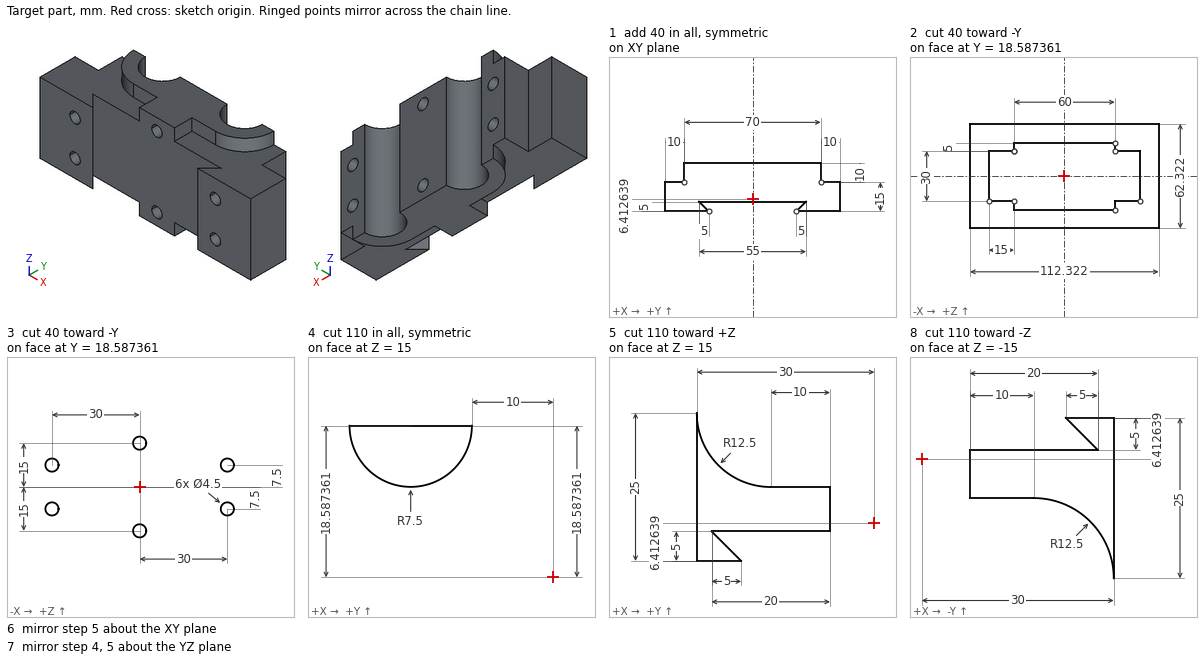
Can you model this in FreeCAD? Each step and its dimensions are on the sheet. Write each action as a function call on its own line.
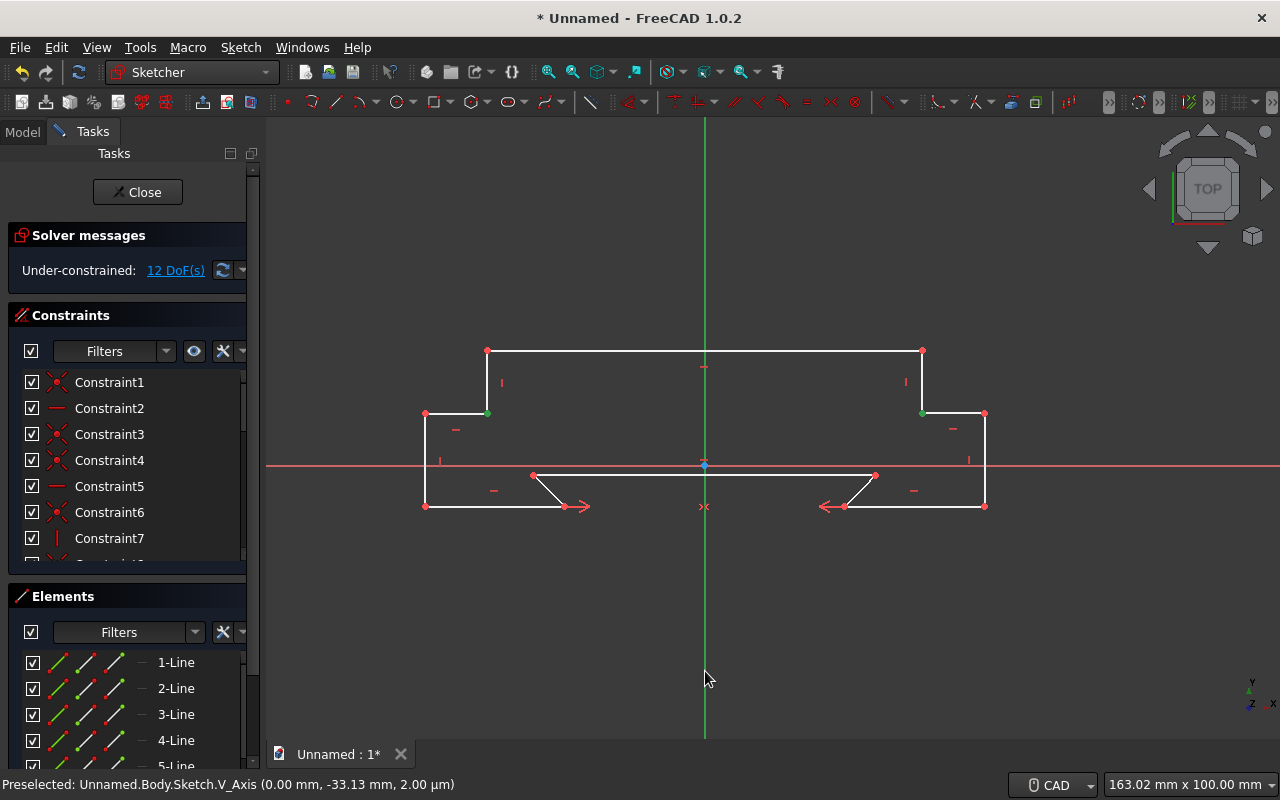
key(s)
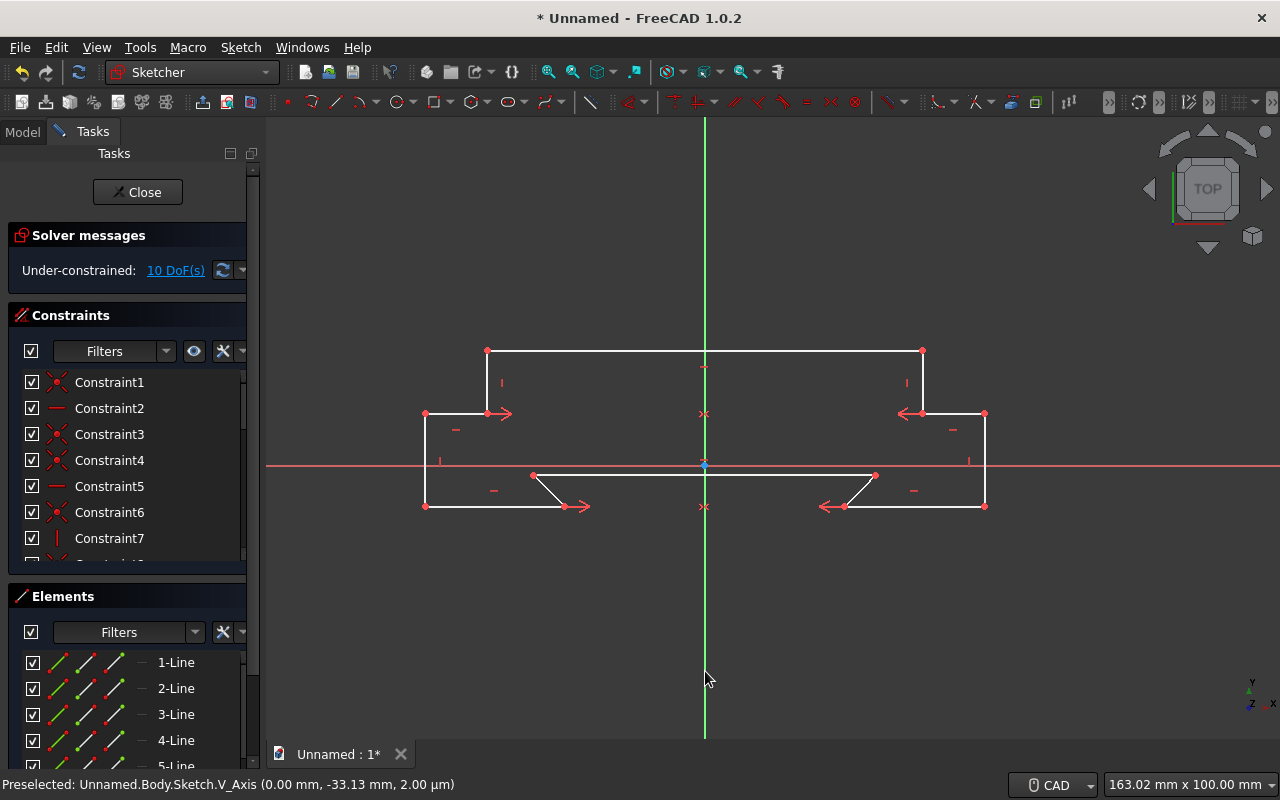
key(d)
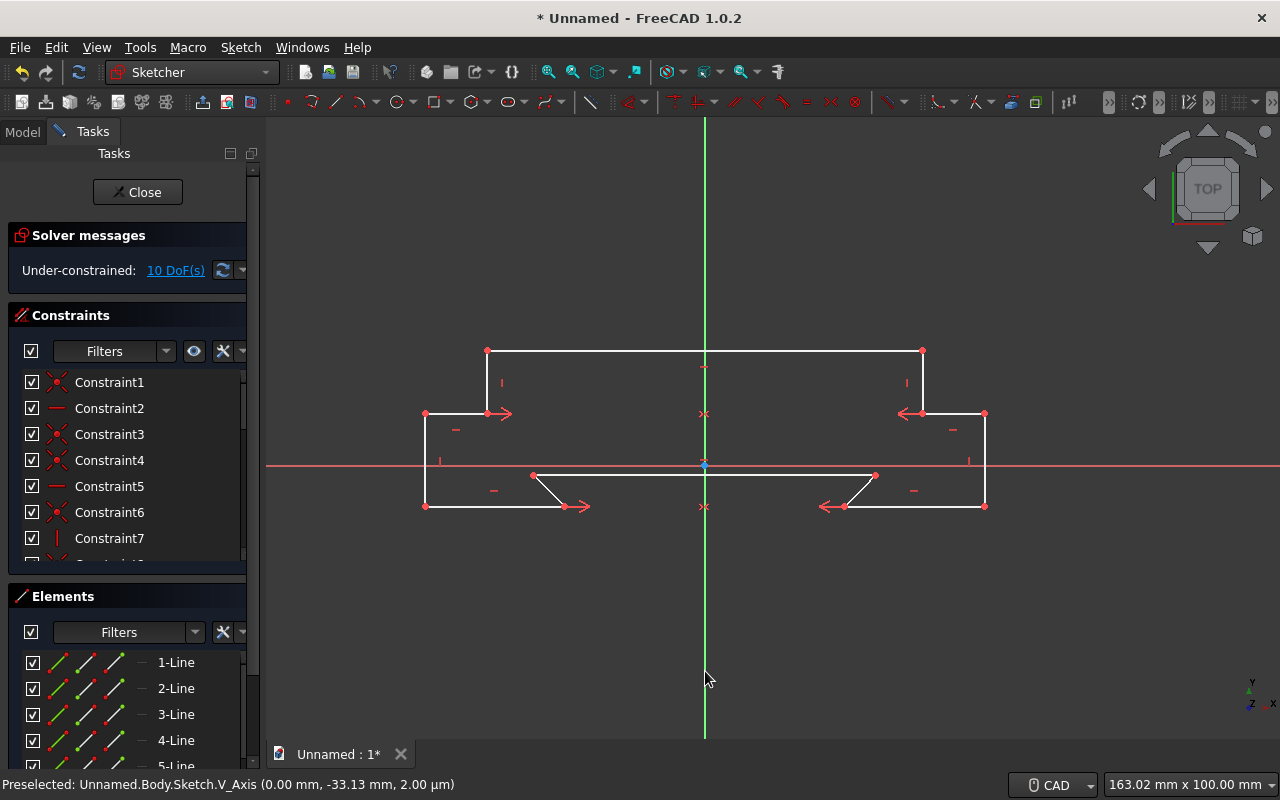
scroll(636, 475, up, 3)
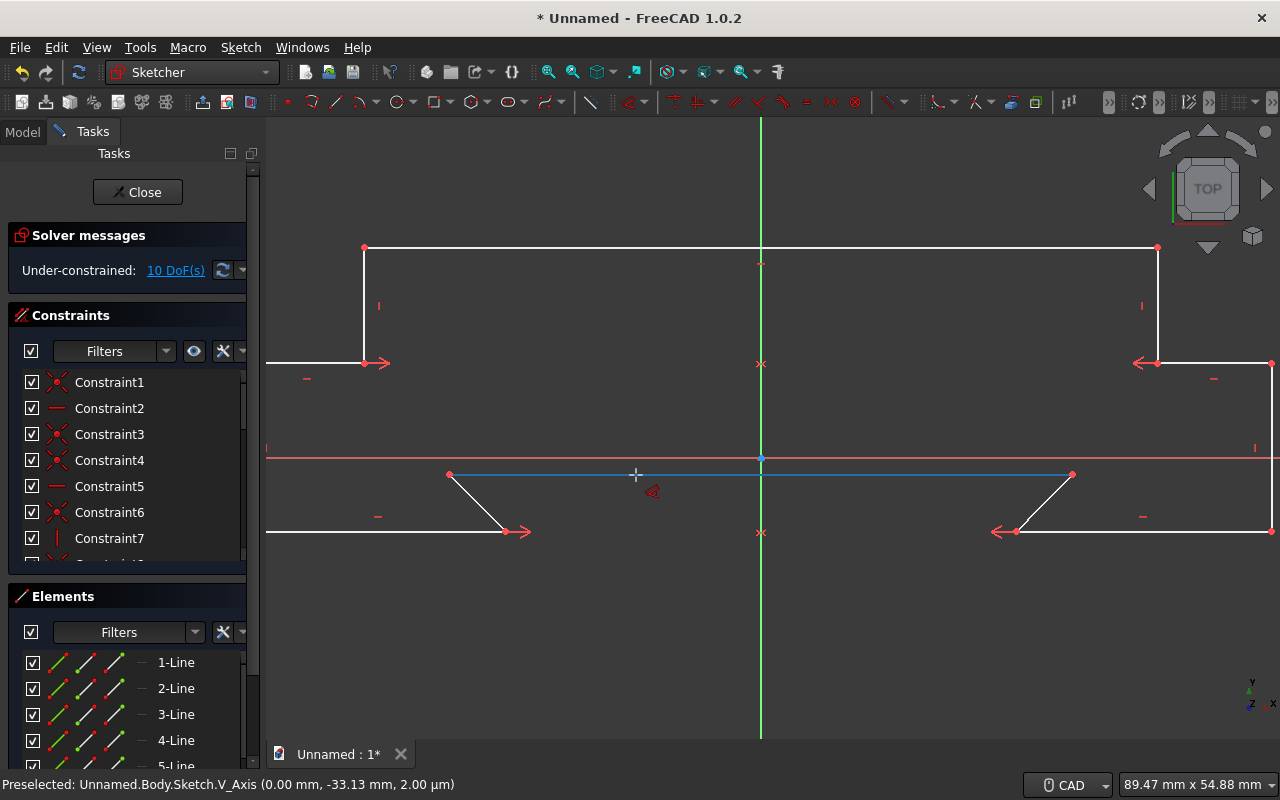
click(637, 475)
click(618, 509)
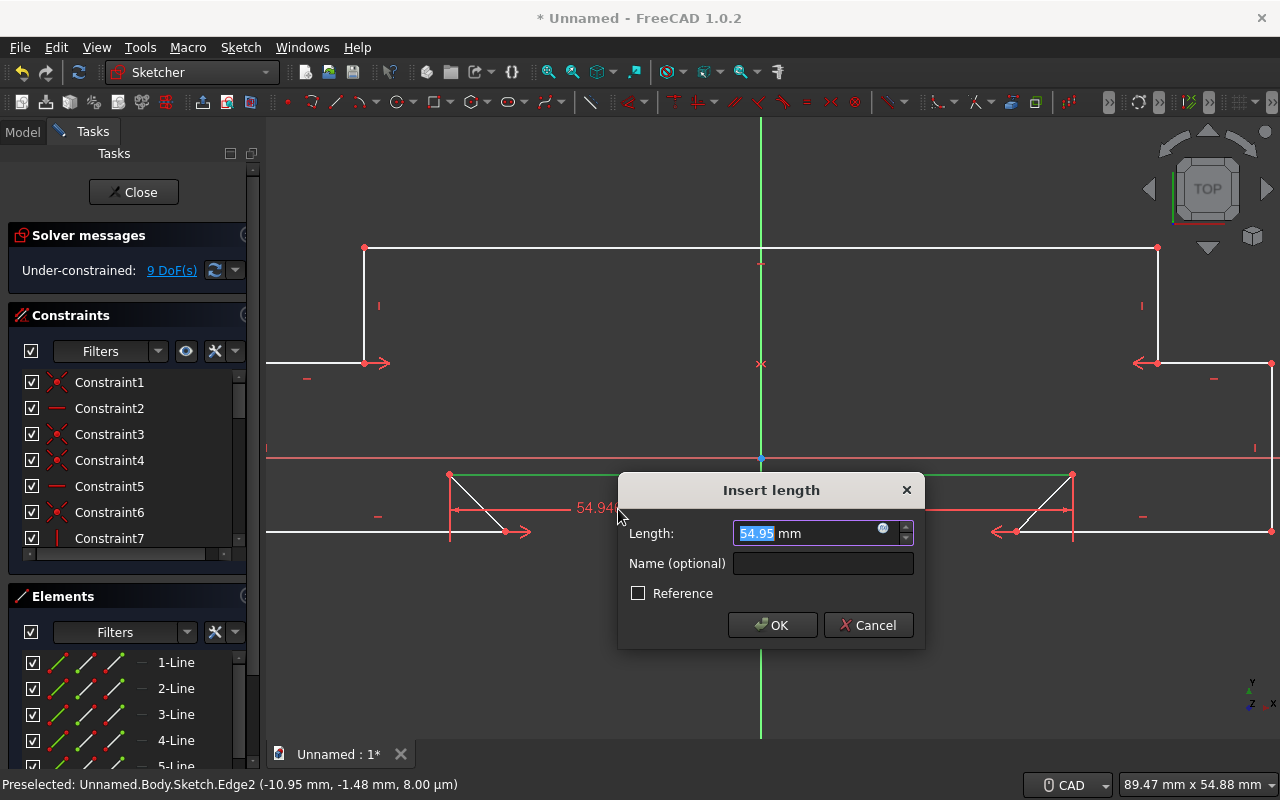
text(55)
key(Return)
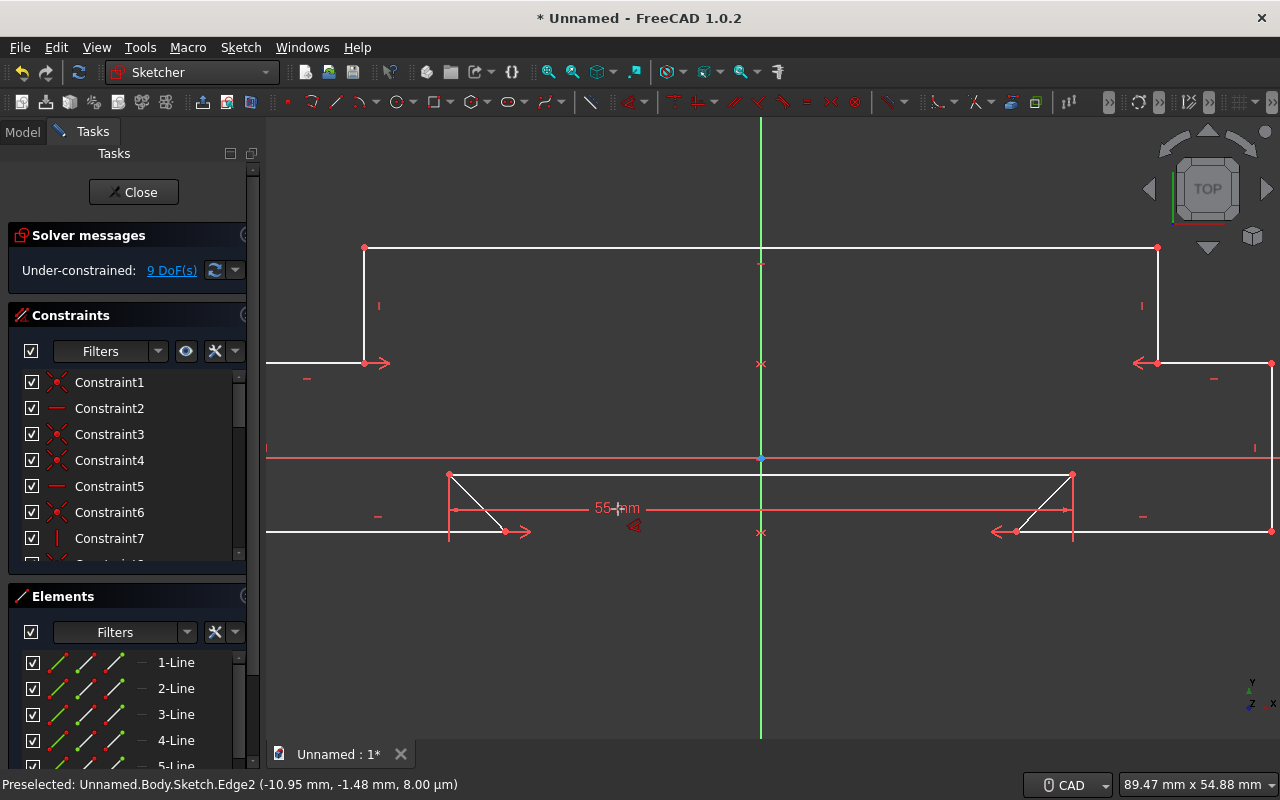
scroll(636, 475, down, 3)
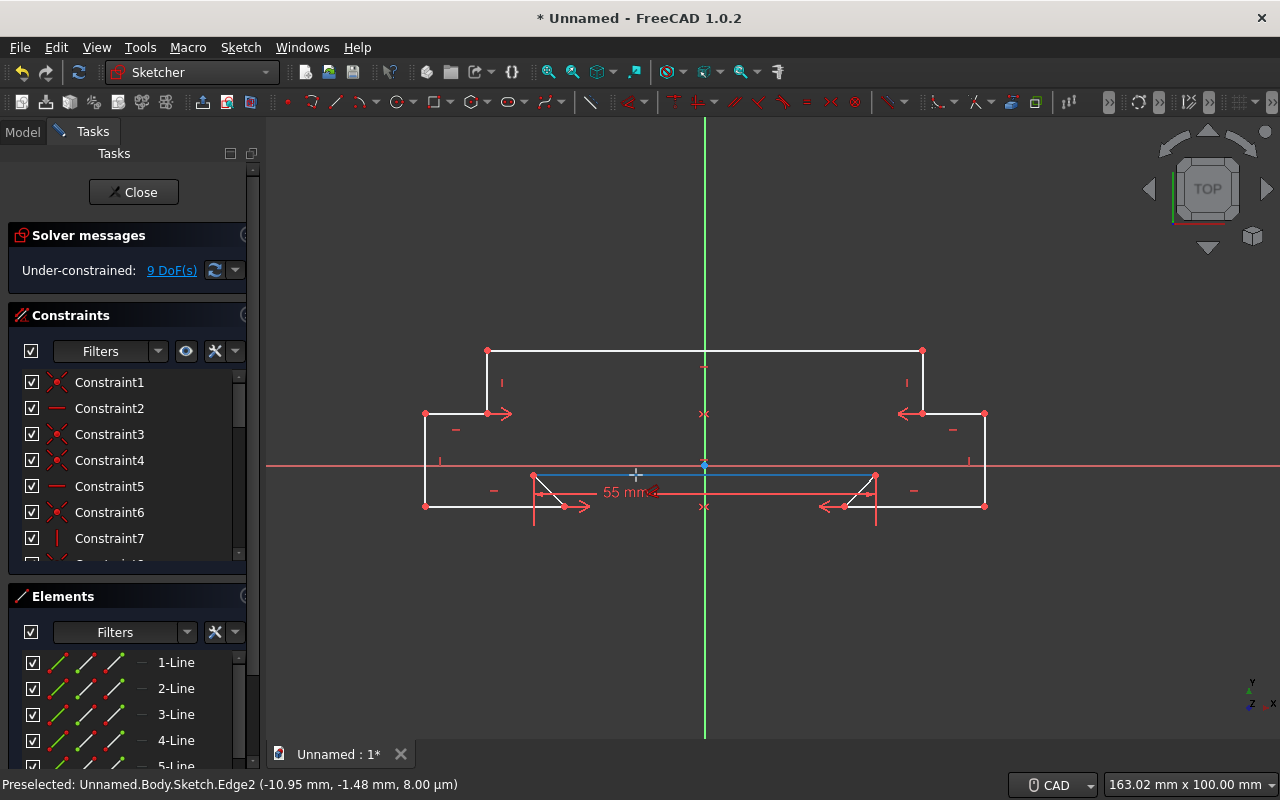
click(985, 479)
click(1019, 439)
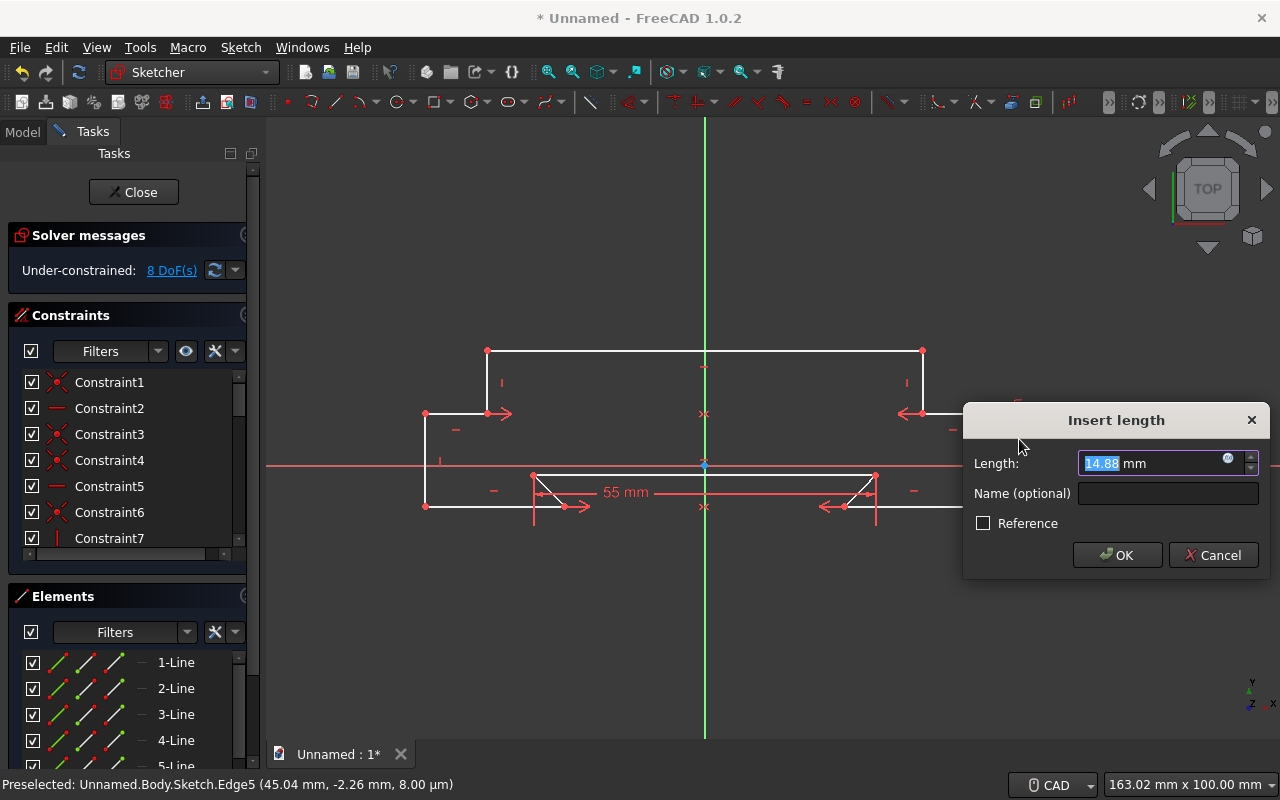
text(15)
key(Return)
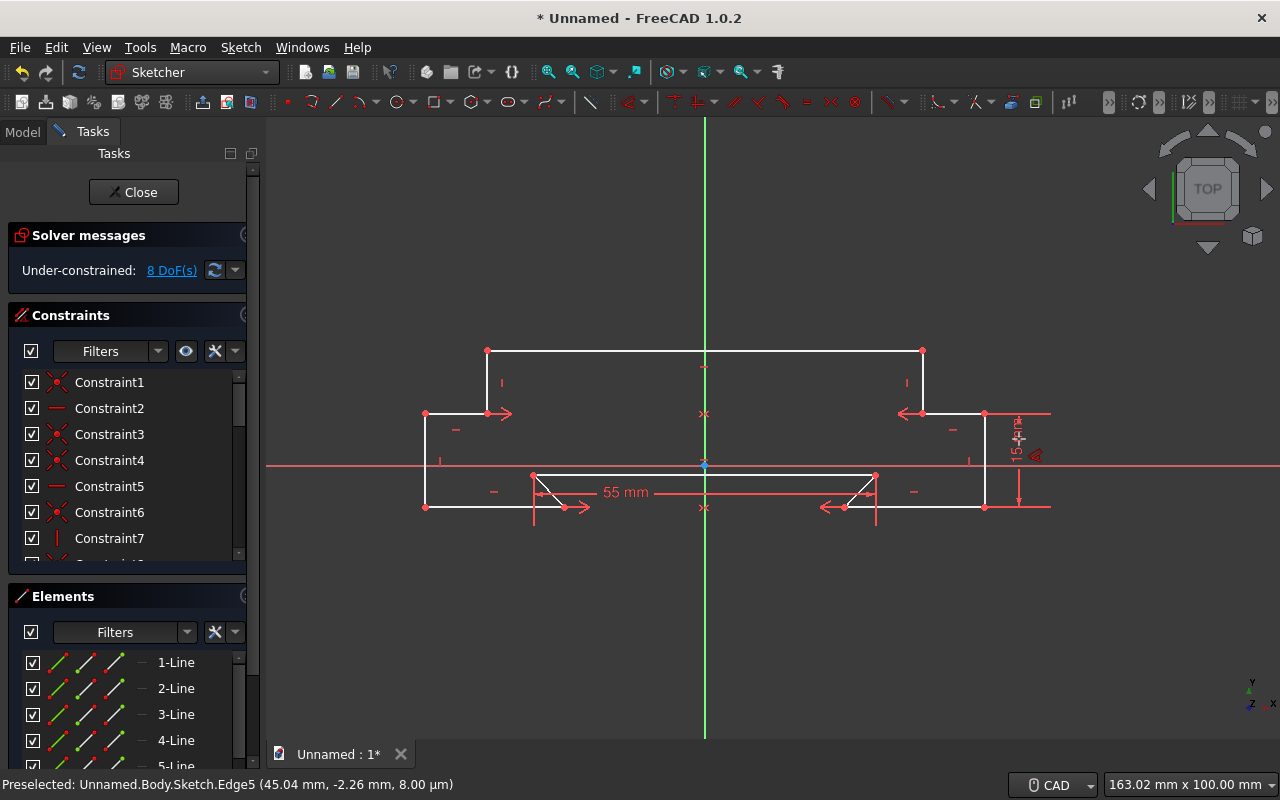
click(966, 414)
click(954, 380)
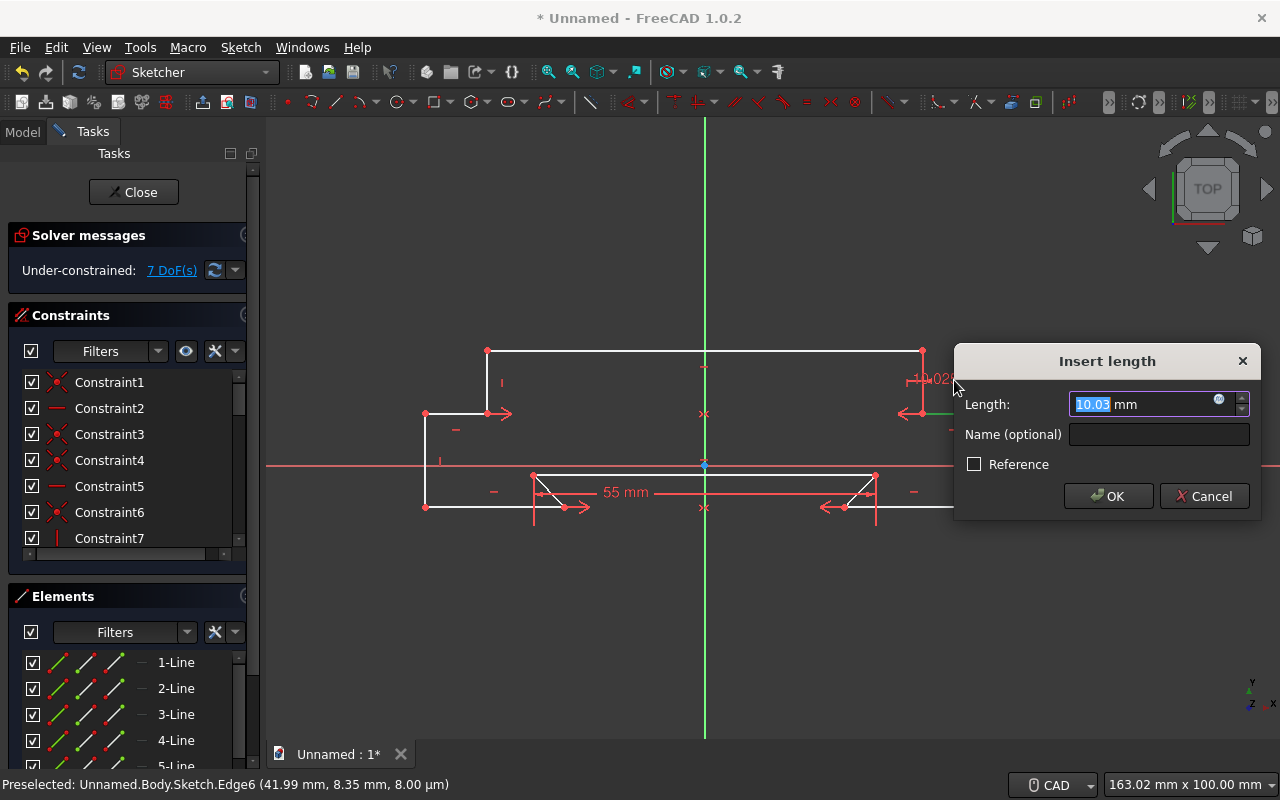
text(10)
key(Return)